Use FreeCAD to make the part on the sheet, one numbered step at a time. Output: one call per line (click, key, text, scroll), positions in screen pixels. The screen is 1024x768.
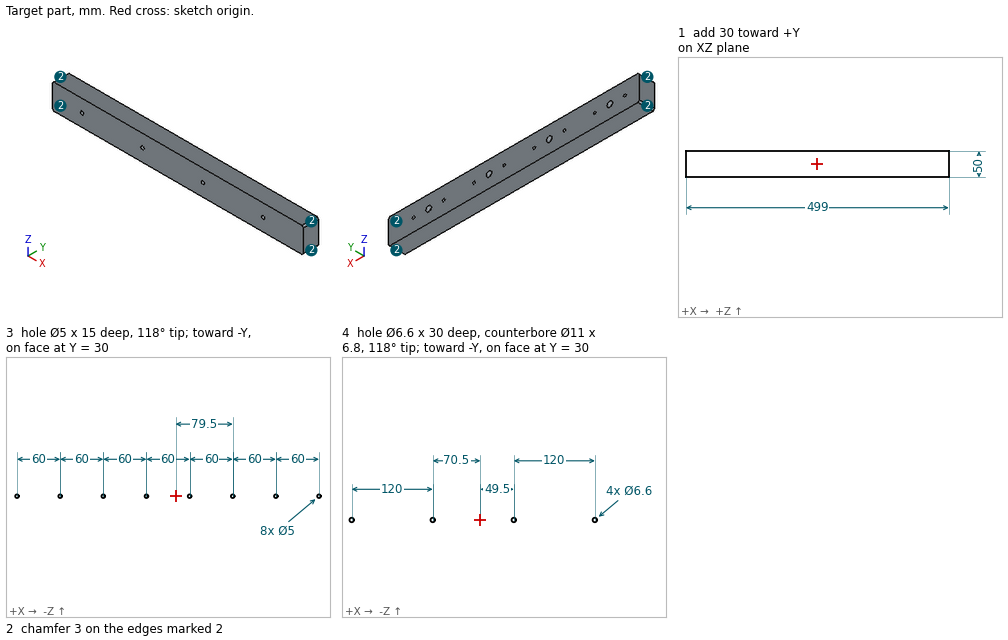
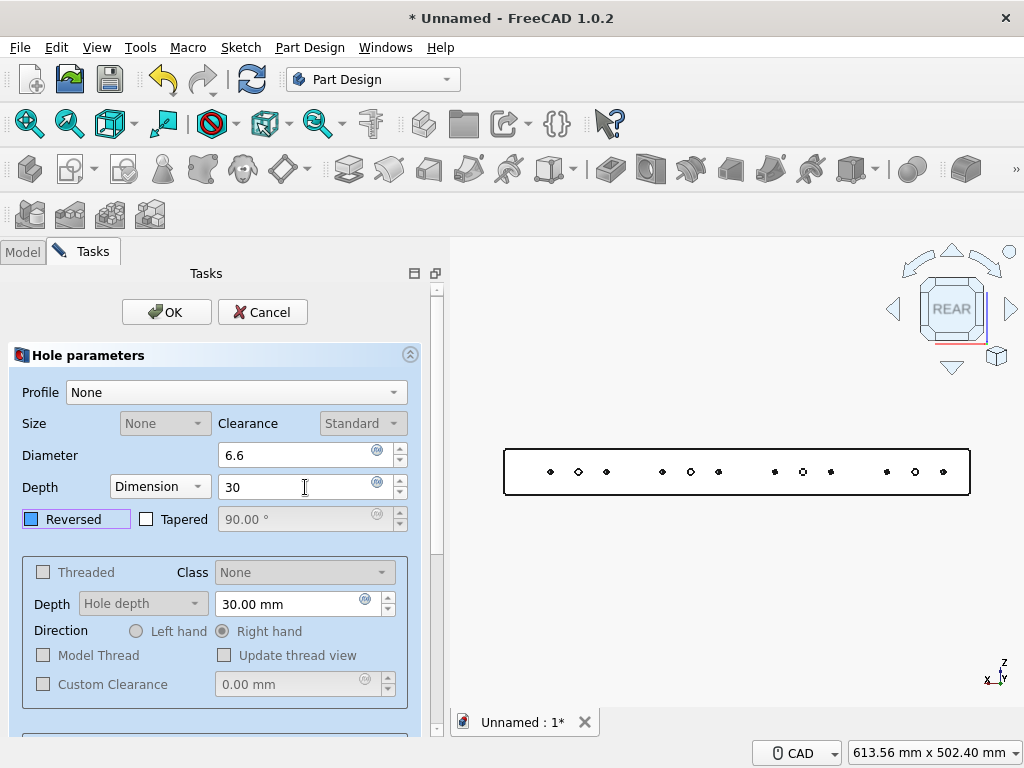
scroll(437, 510, down, 2)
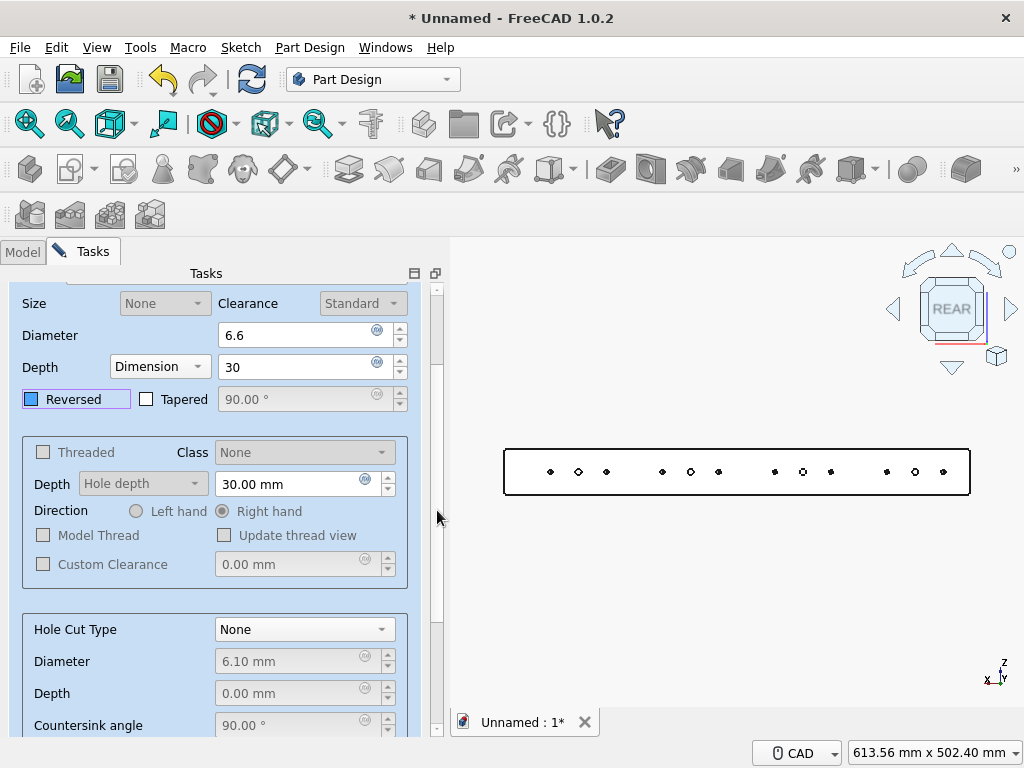
click(306, 630)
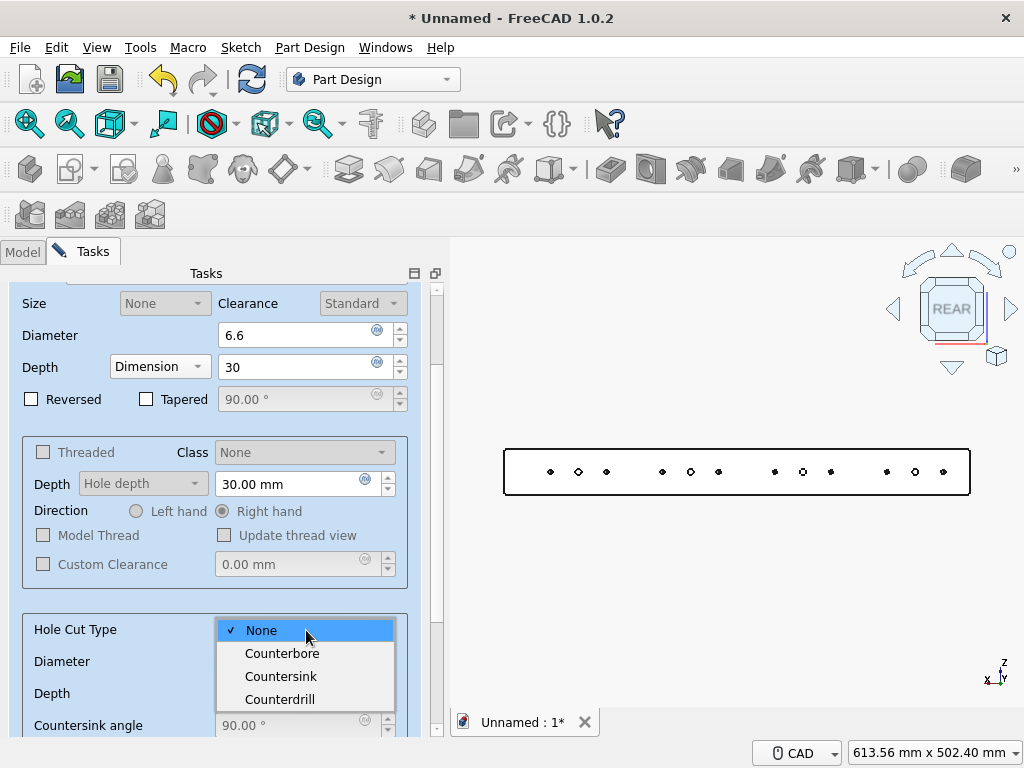
click(304, 654)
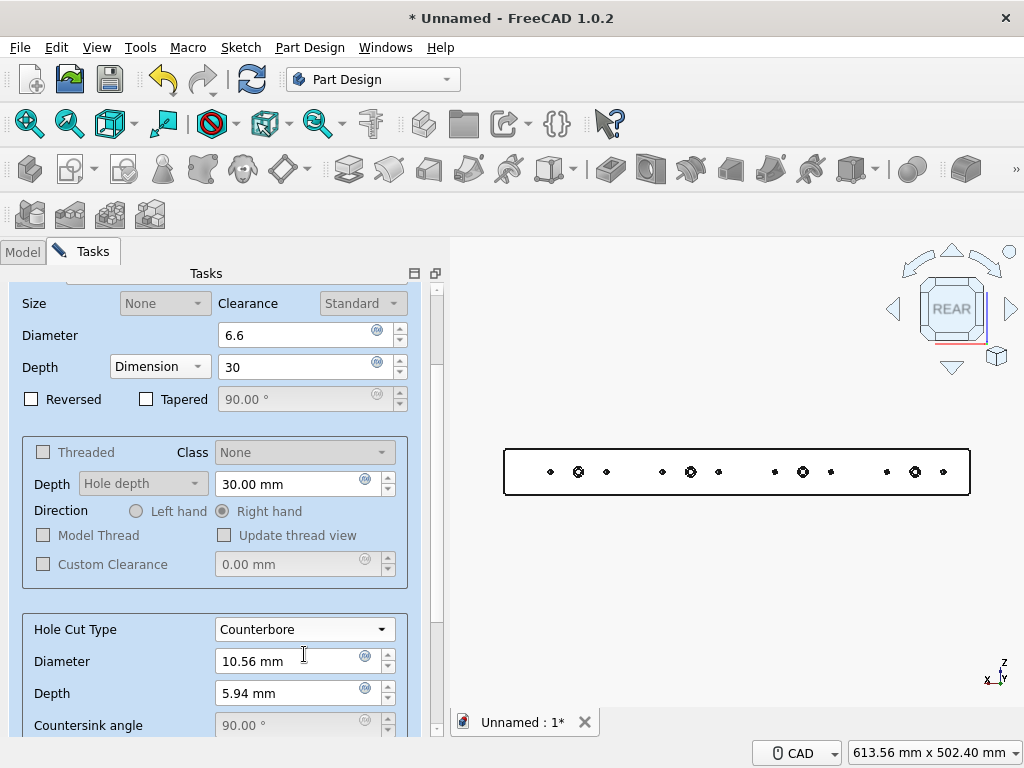
triple_click(298, 661)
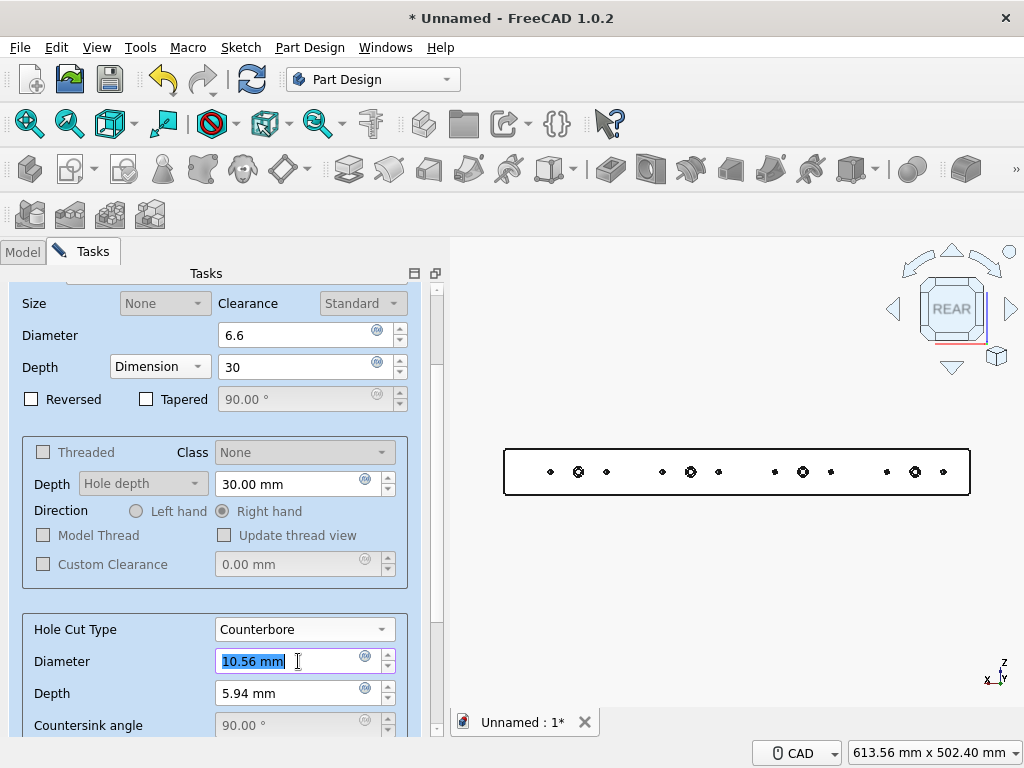
text(11)
key(Tab)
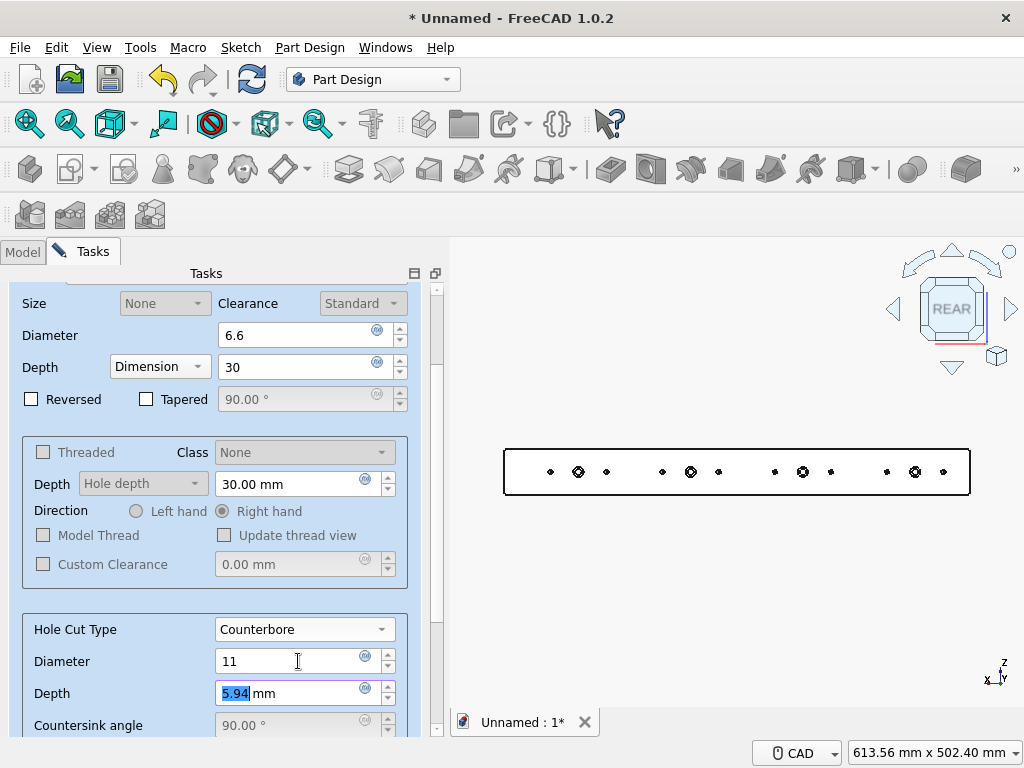
text(6.8)
key(Tab)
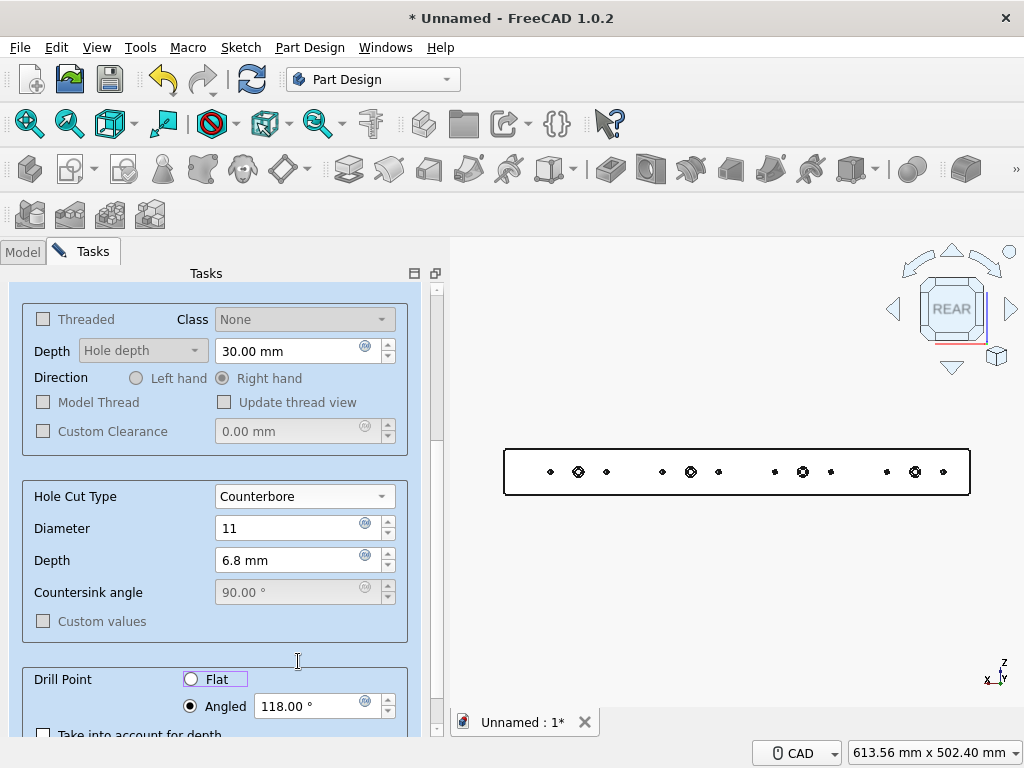
scroll(437, 510, up, 5)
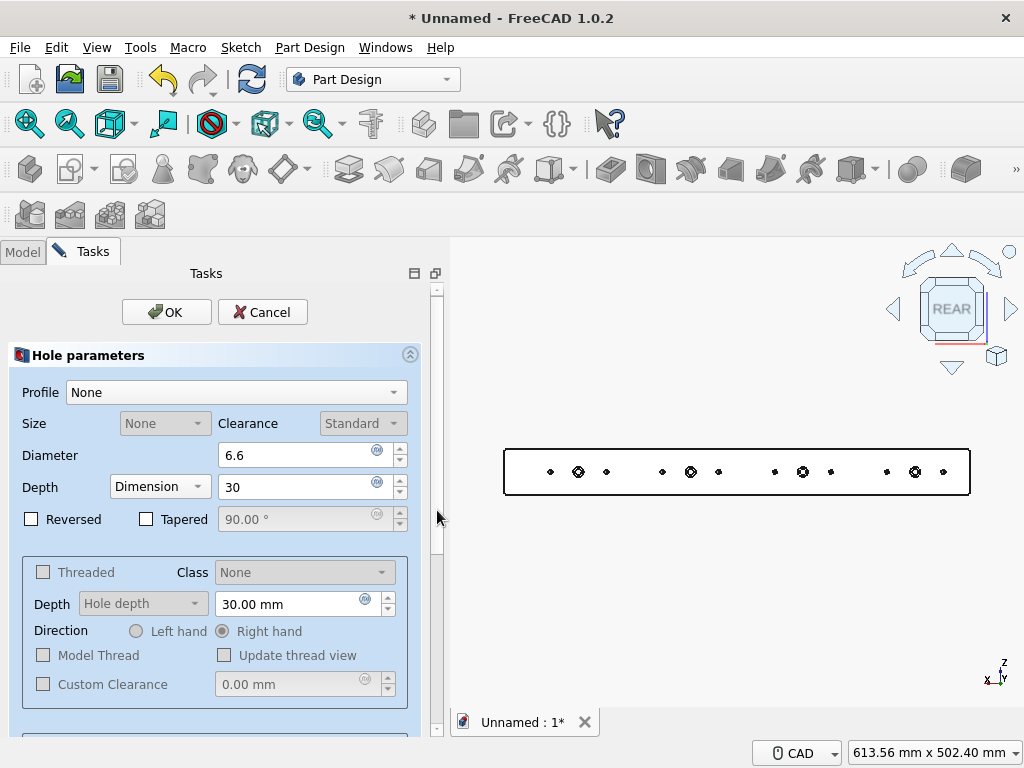
click(167, 312)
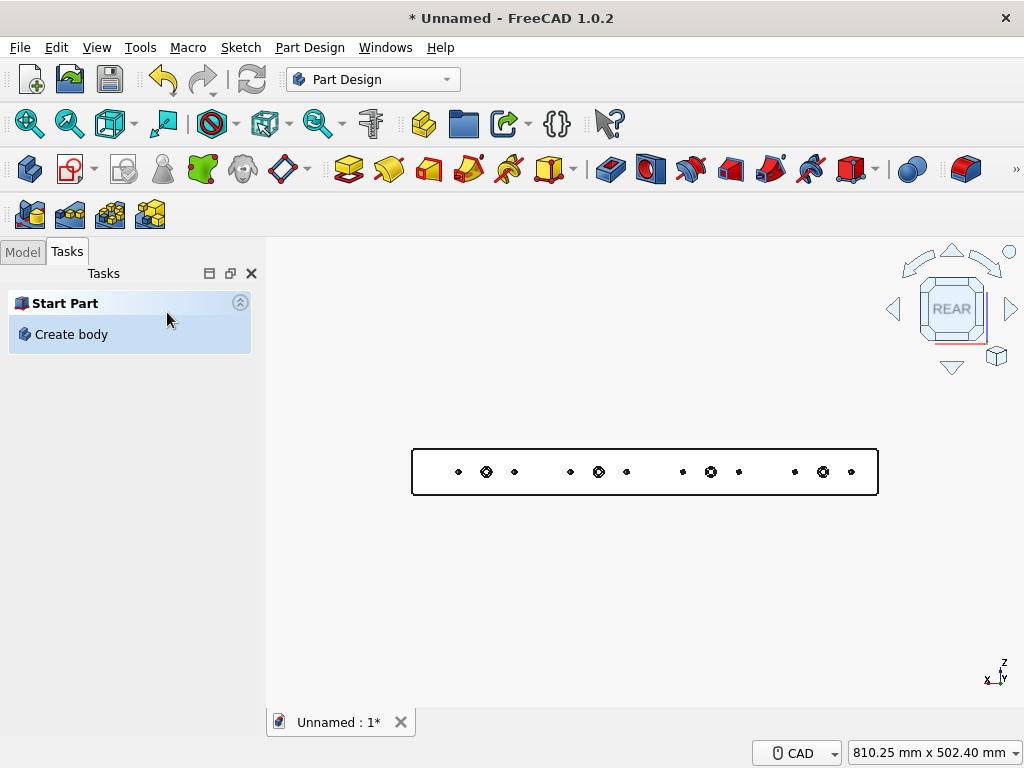
key(0)